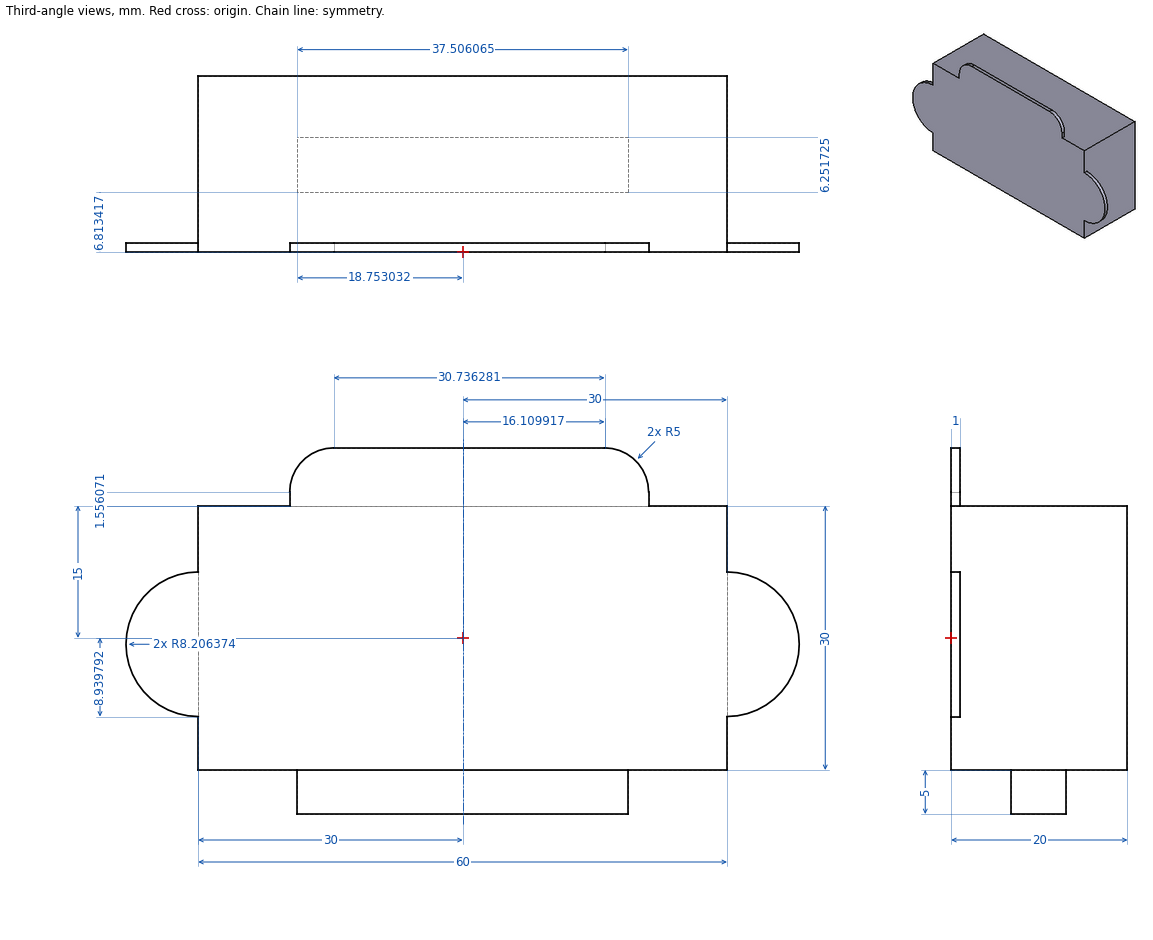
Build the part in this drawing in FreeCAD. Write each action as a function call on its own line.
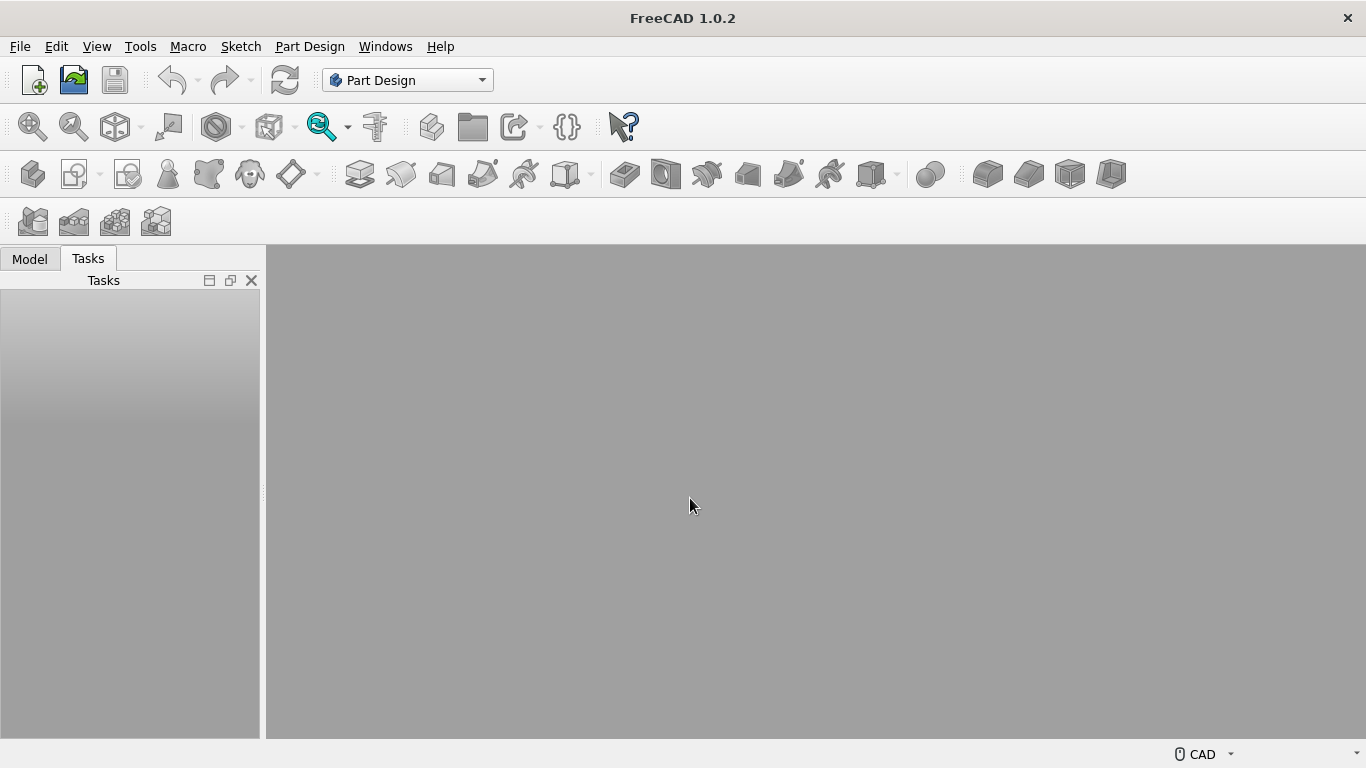
click(33, 80)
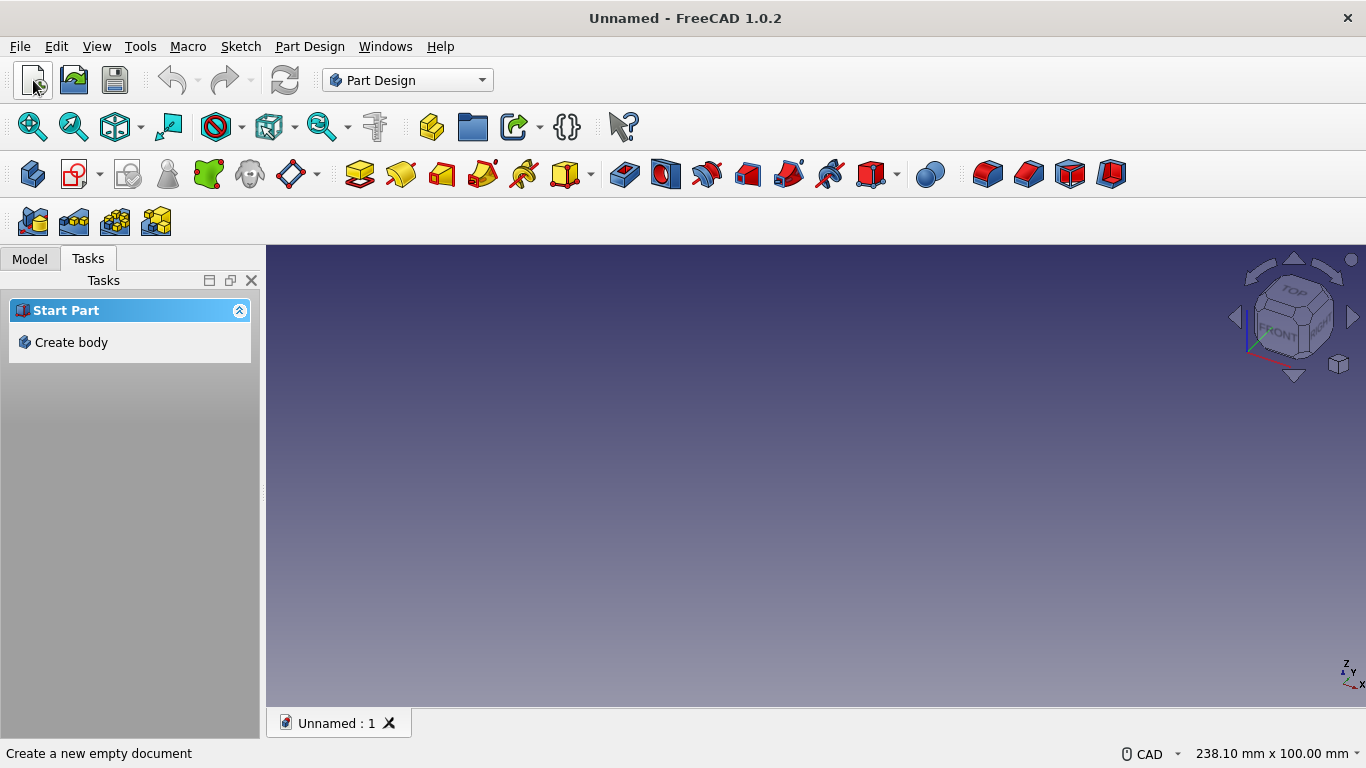
click(74, 174)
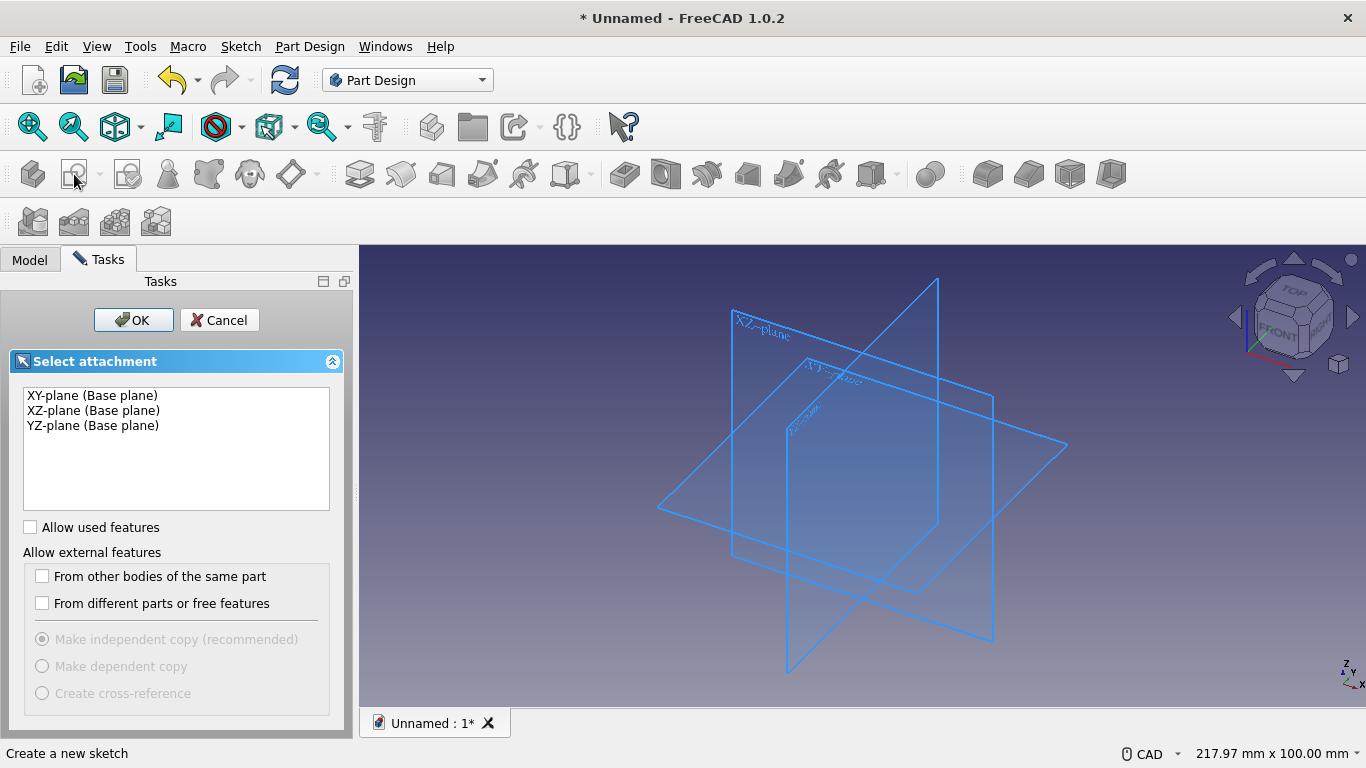
click(84, 410)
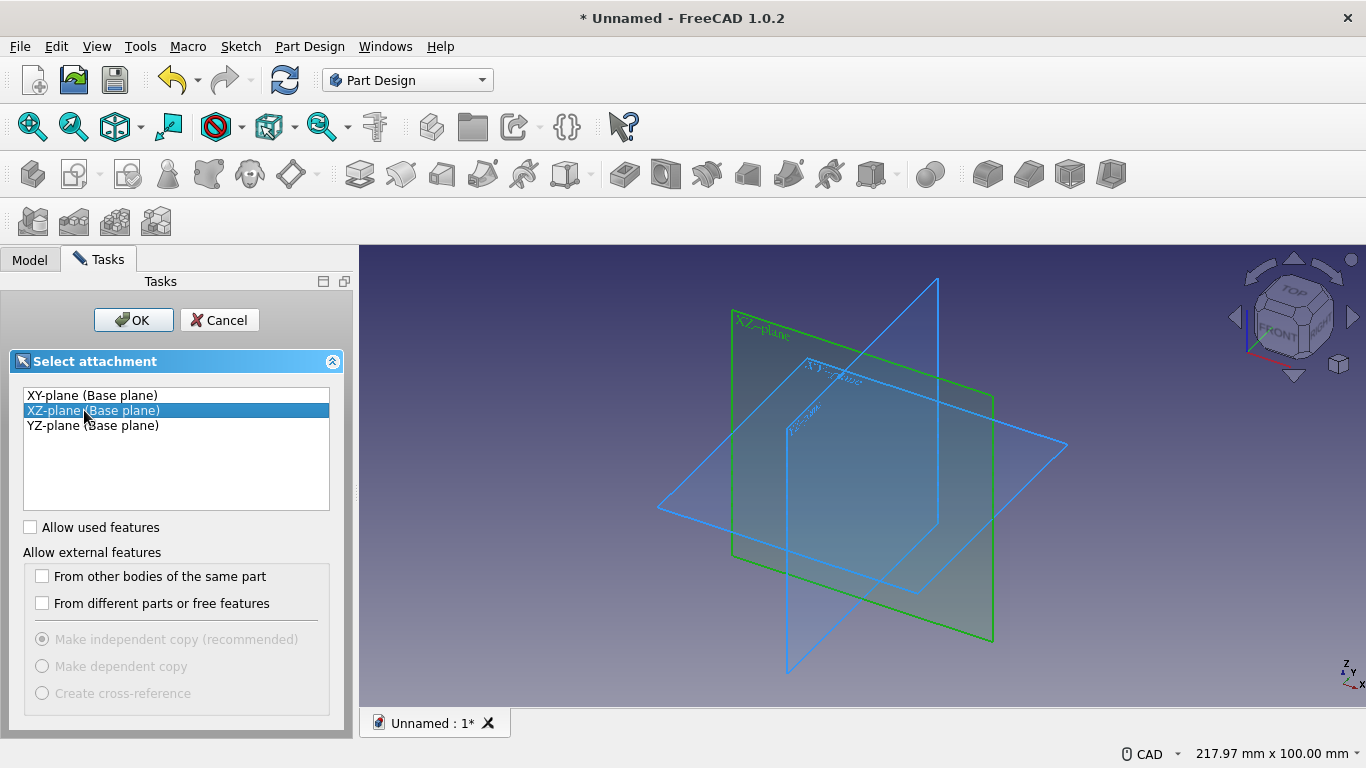
click(134, 320)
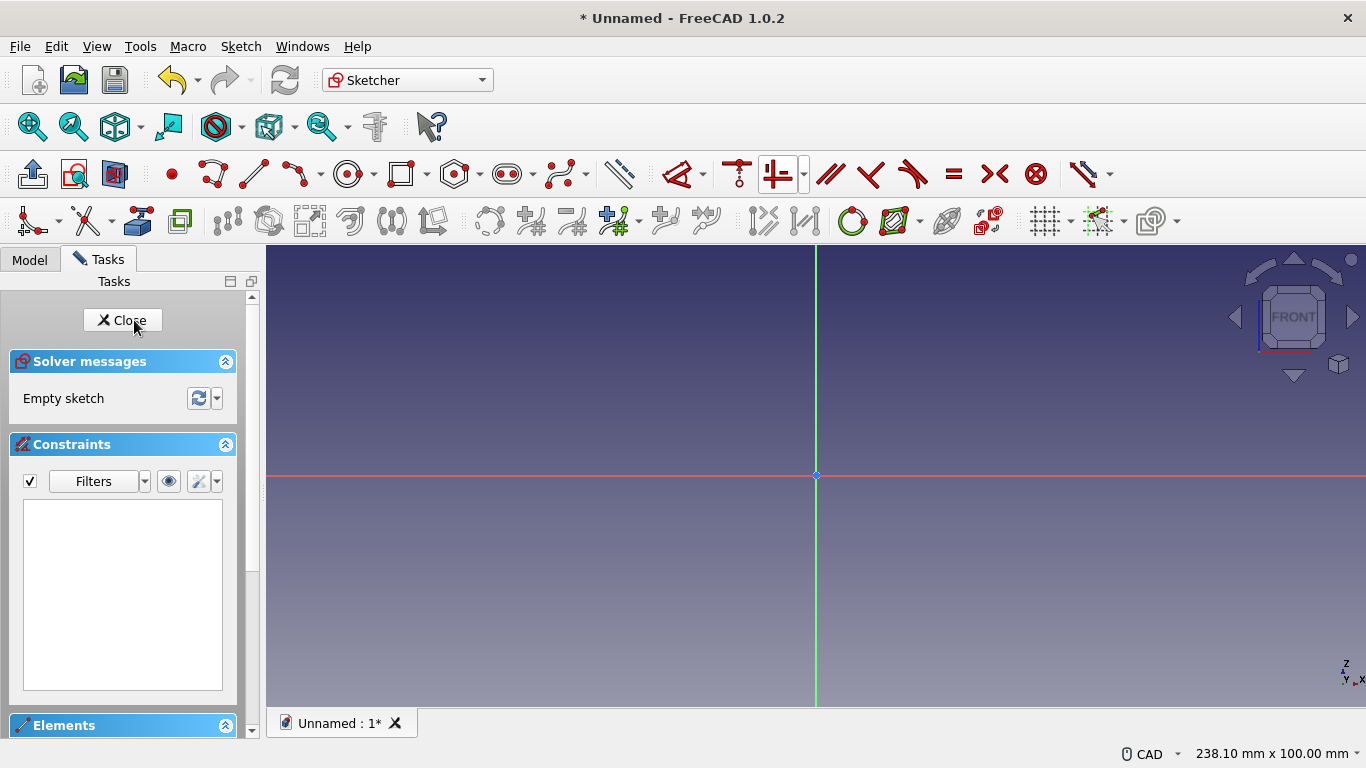
scroll(872, 476, up, 4)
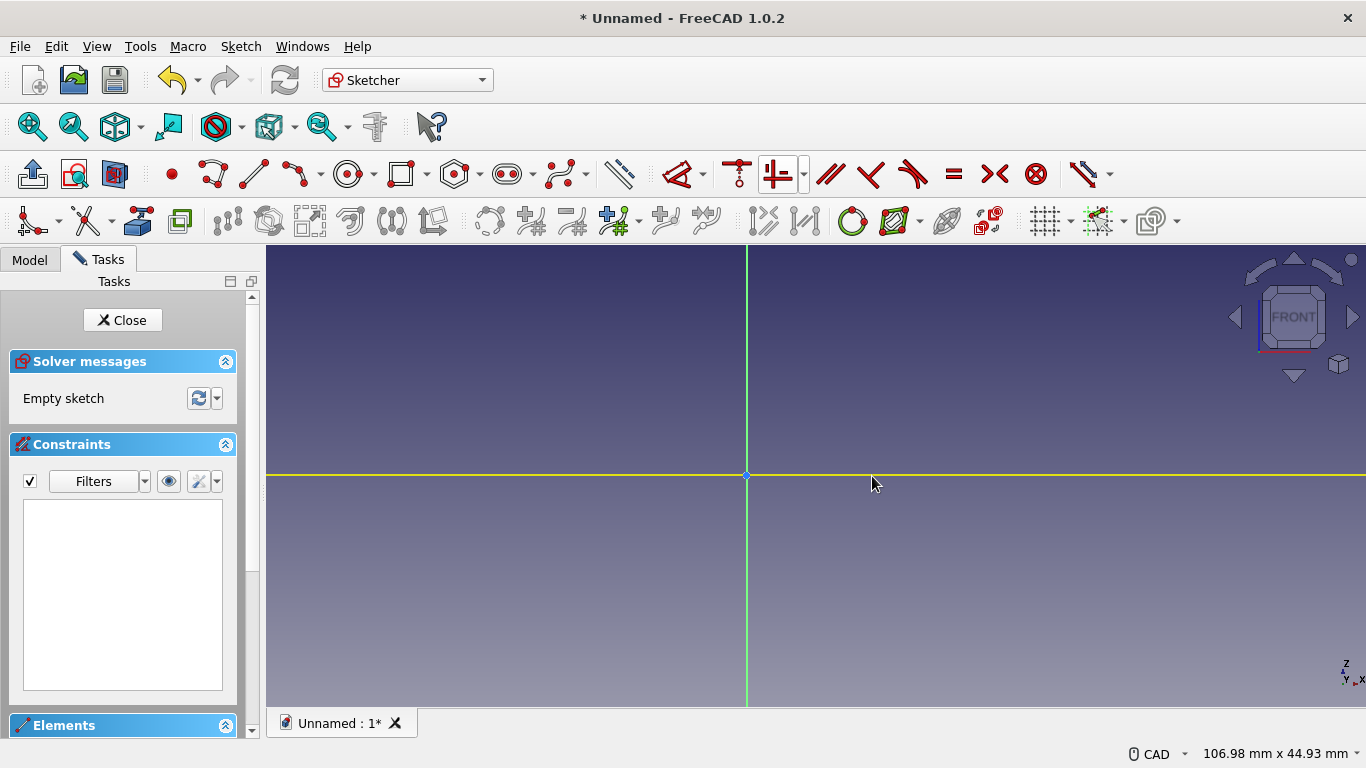
key(g)
key(v)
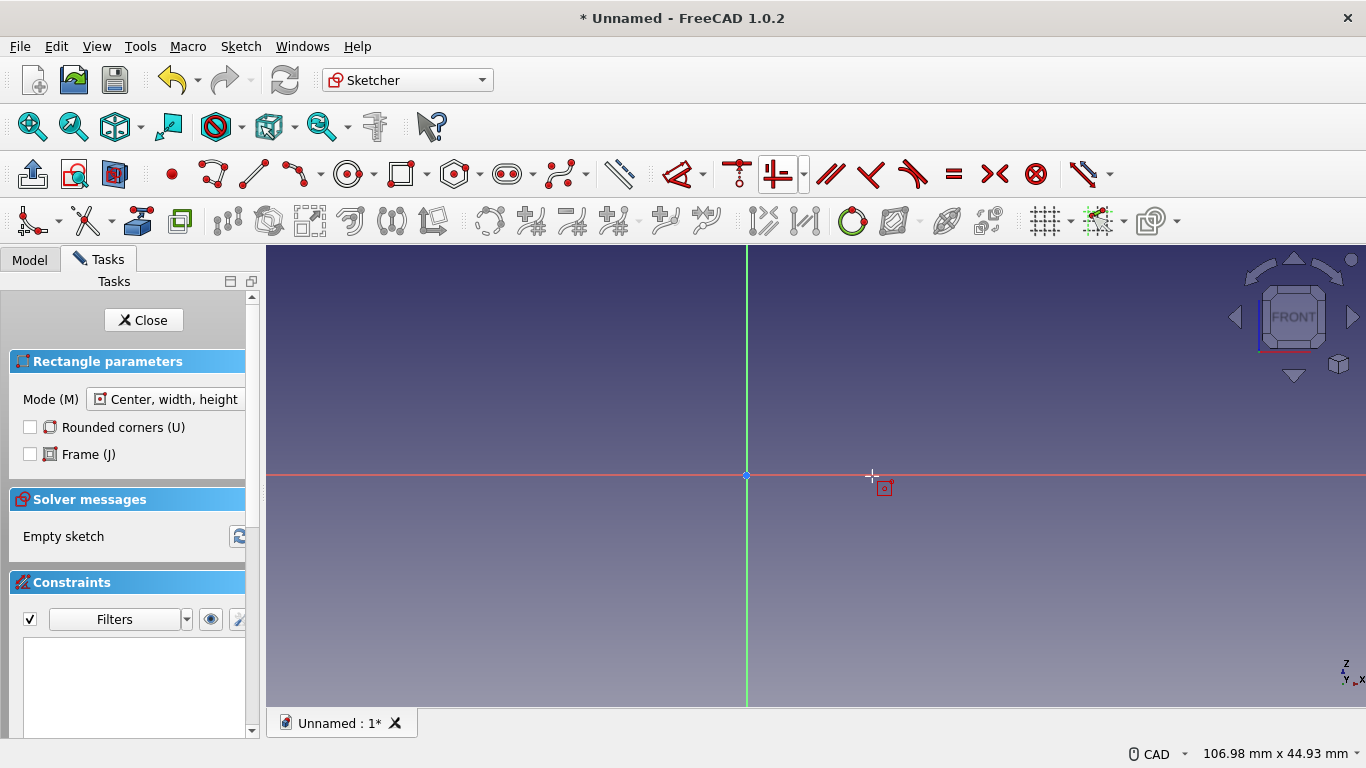
click(747, 475)
move(1055, 321)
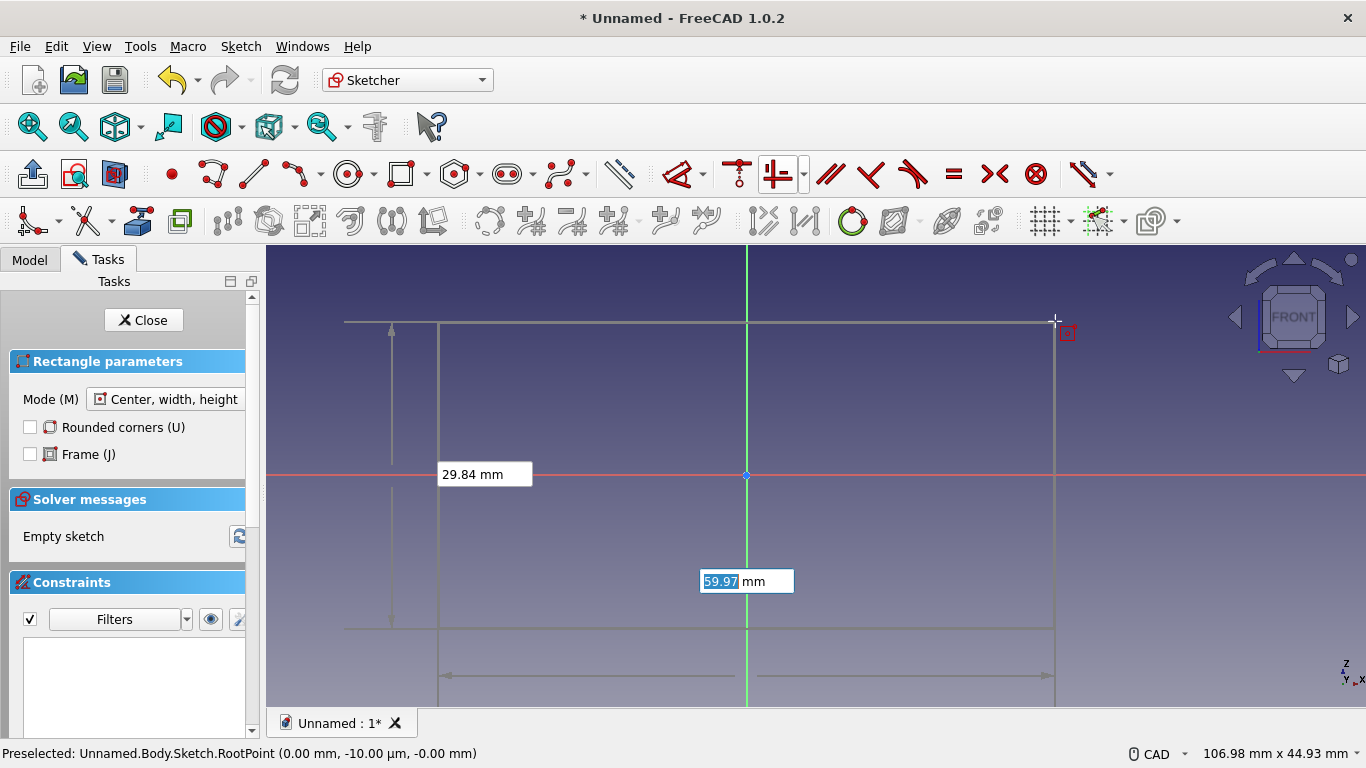
text(60)
key(Tab)
text(30)
key(Return)
key(Escape)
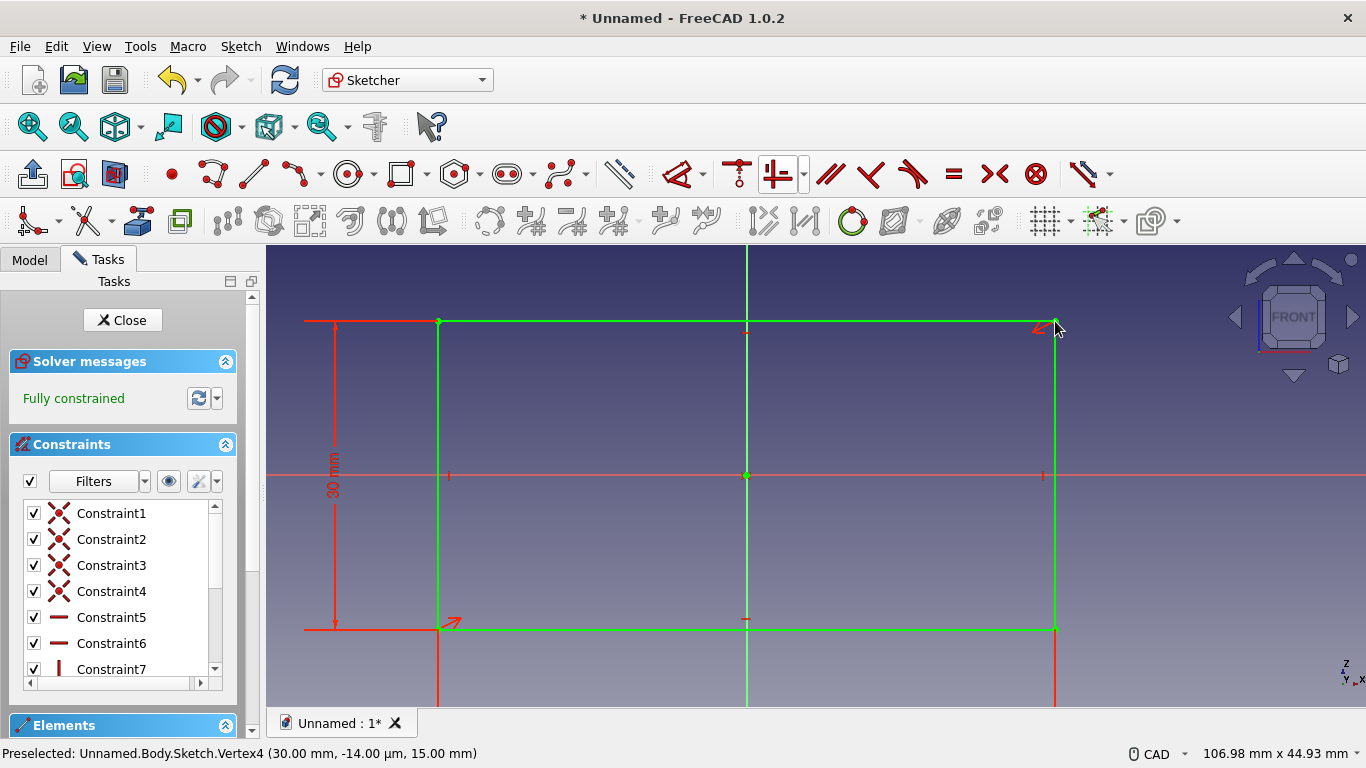
click(123, 320)